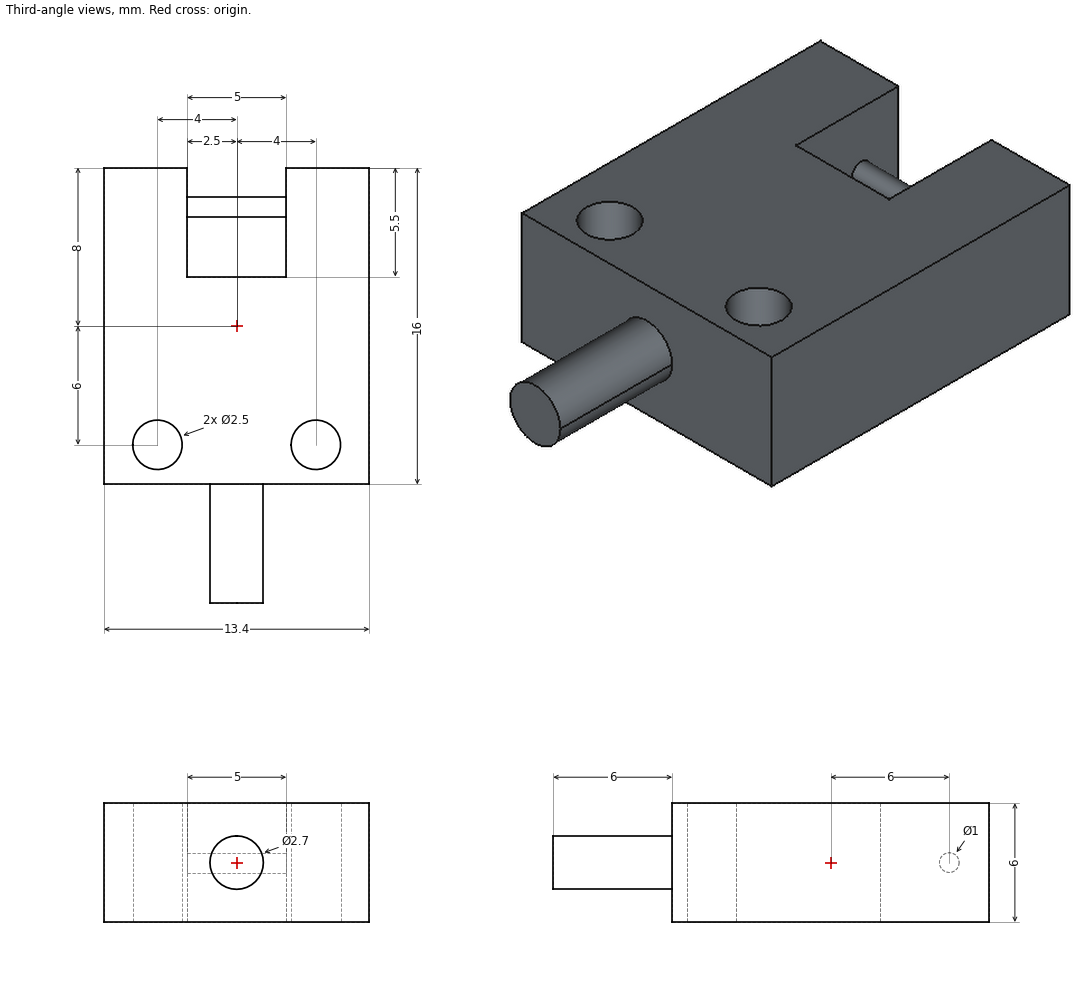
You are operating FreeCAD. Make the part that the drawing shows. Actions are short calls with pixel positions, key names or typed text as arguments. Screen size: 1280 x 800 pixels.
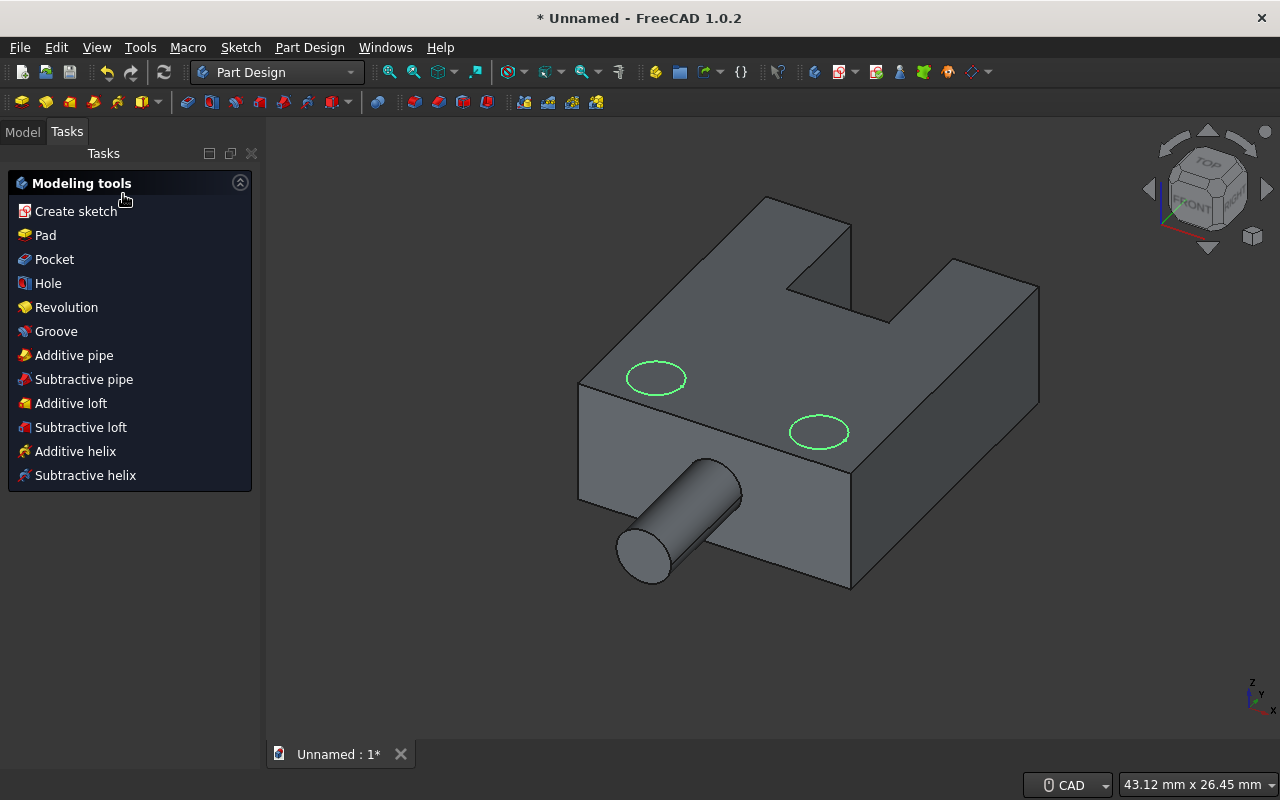
click(188, 102)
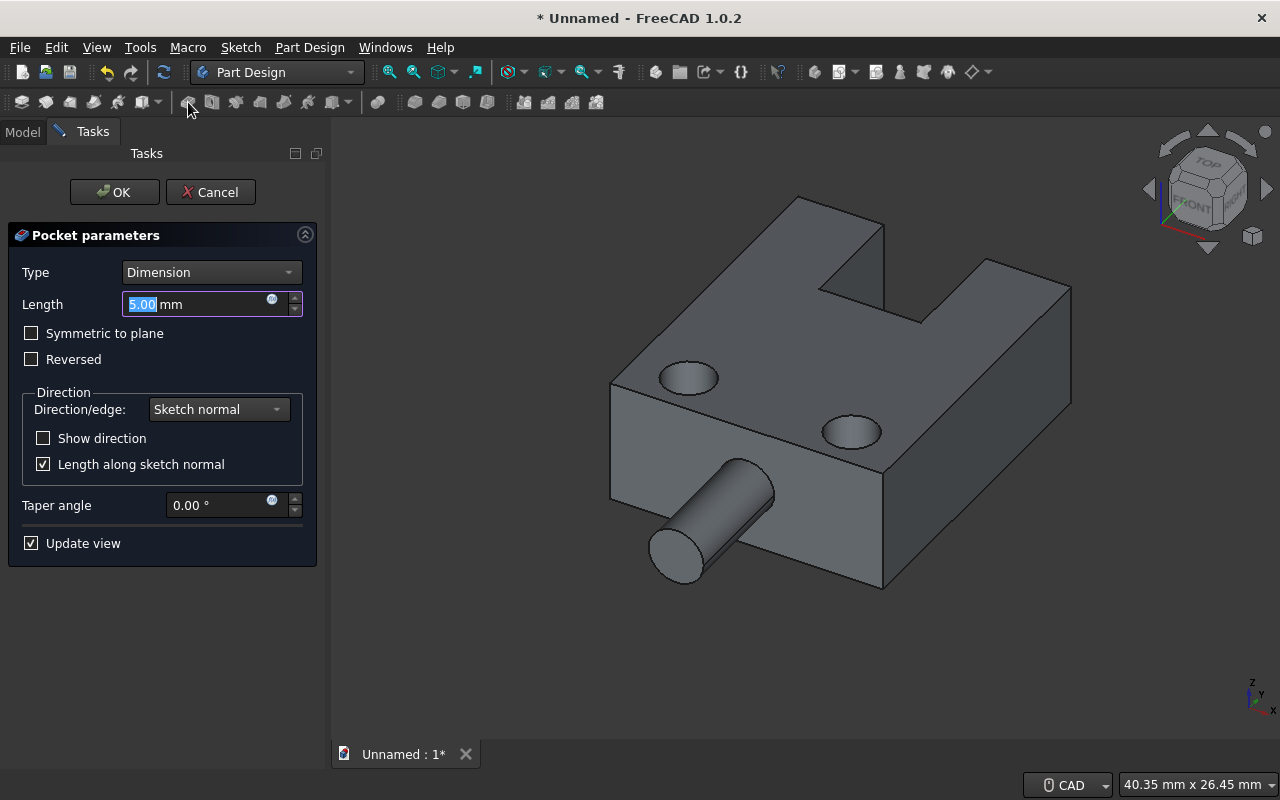
click(212, 272)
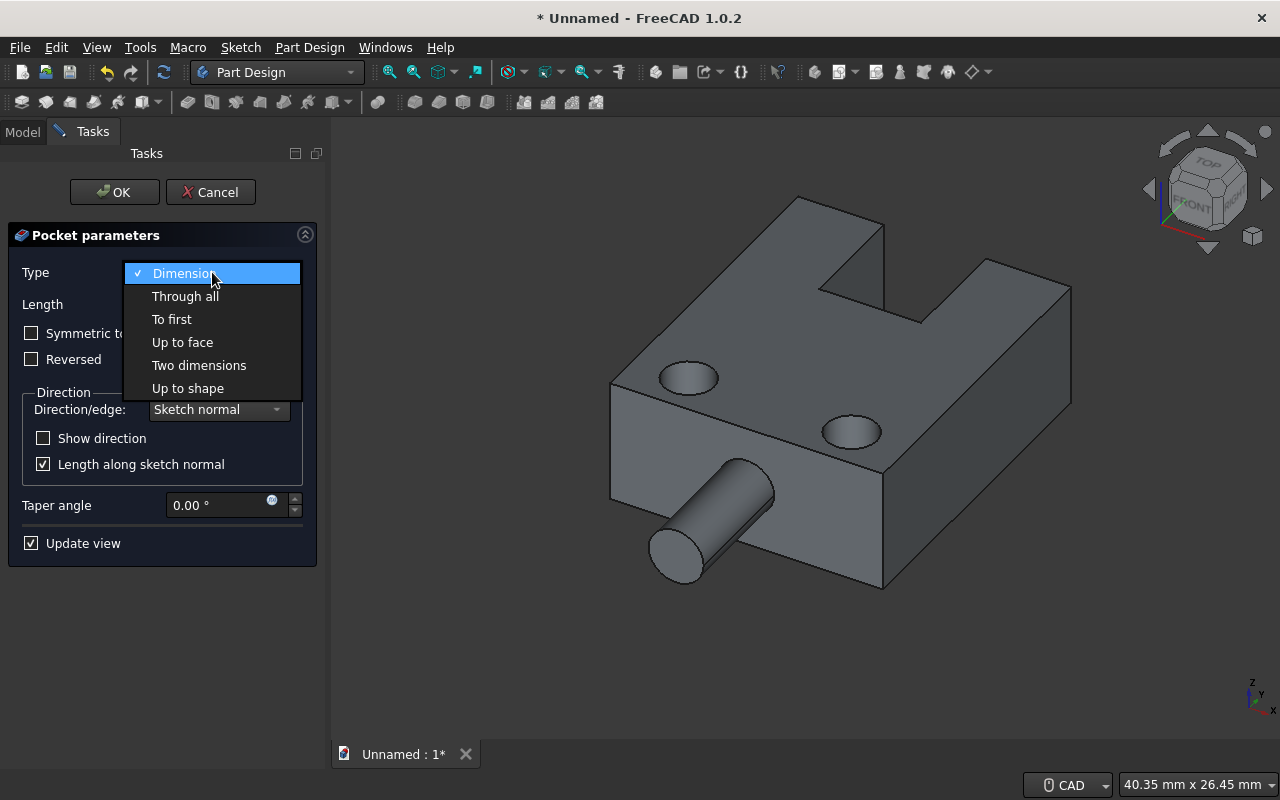
click(212, 296)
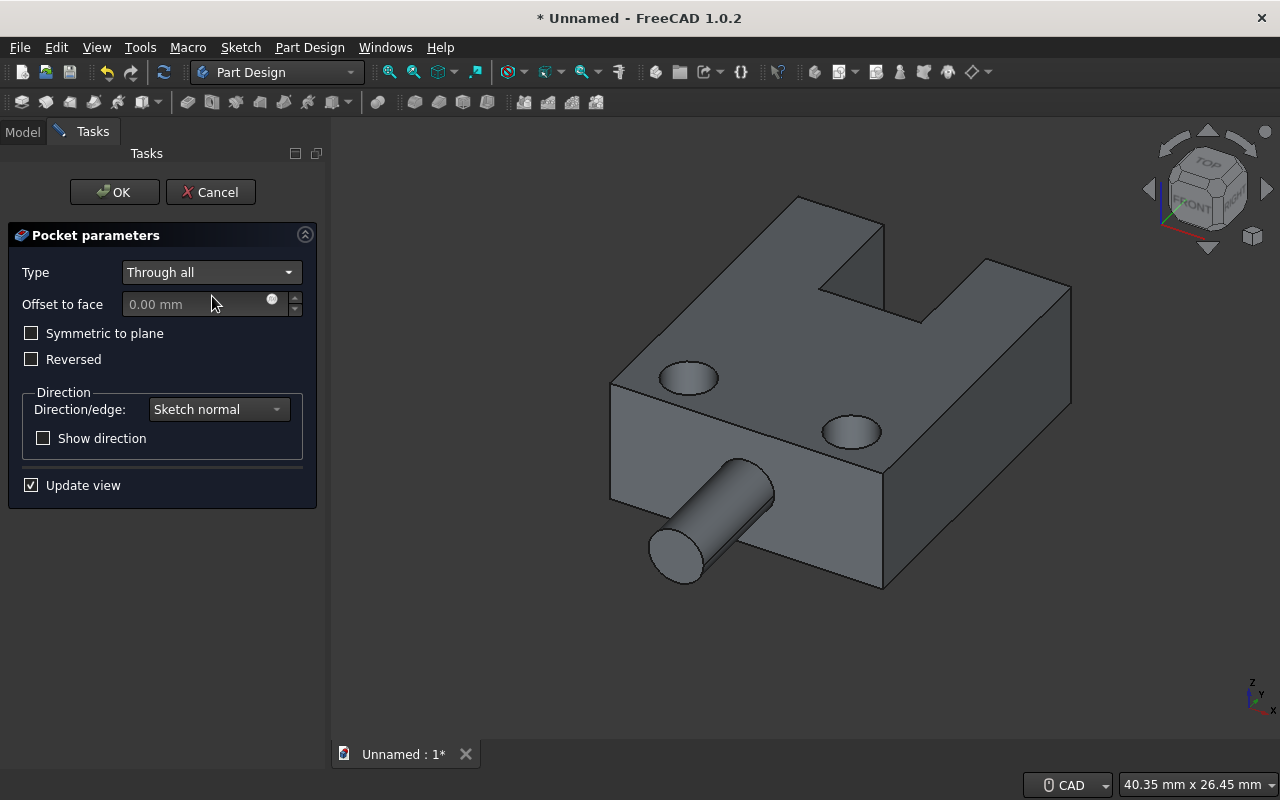
click(115, 192)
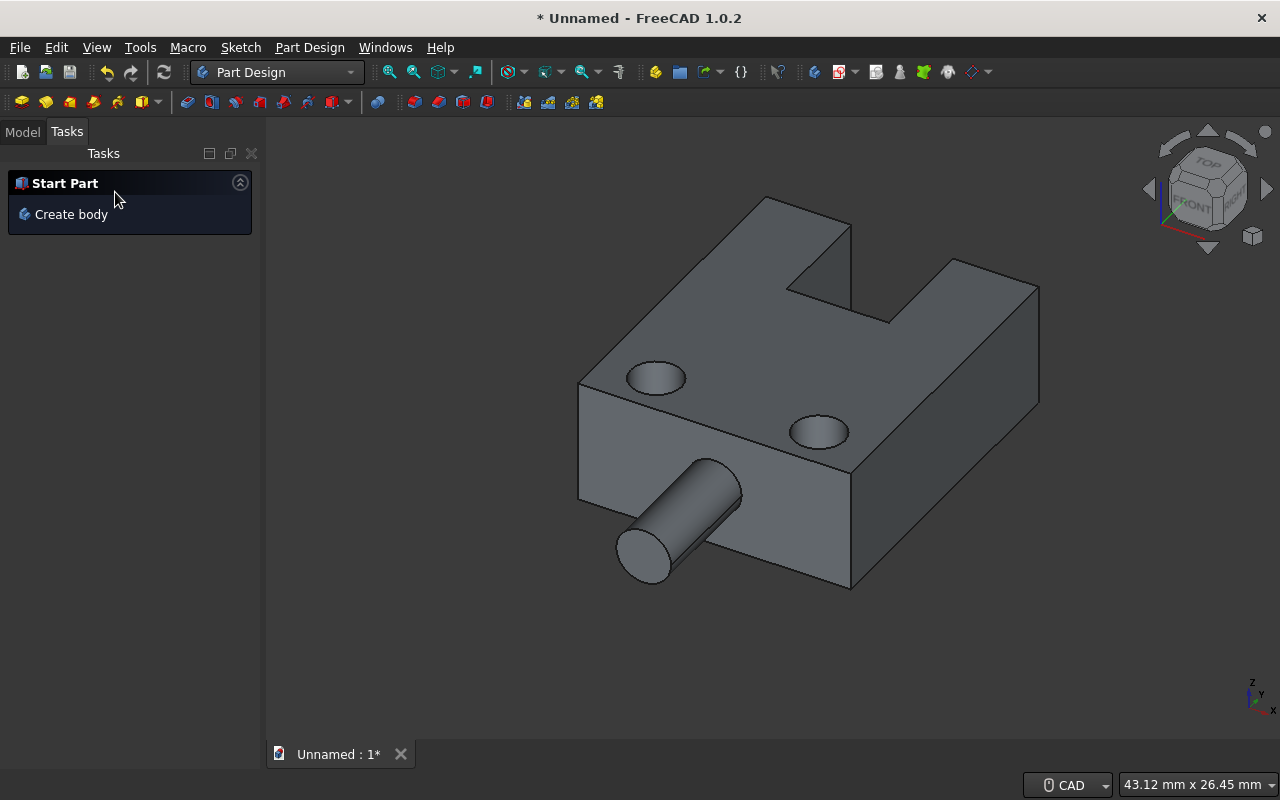
click(23, 131)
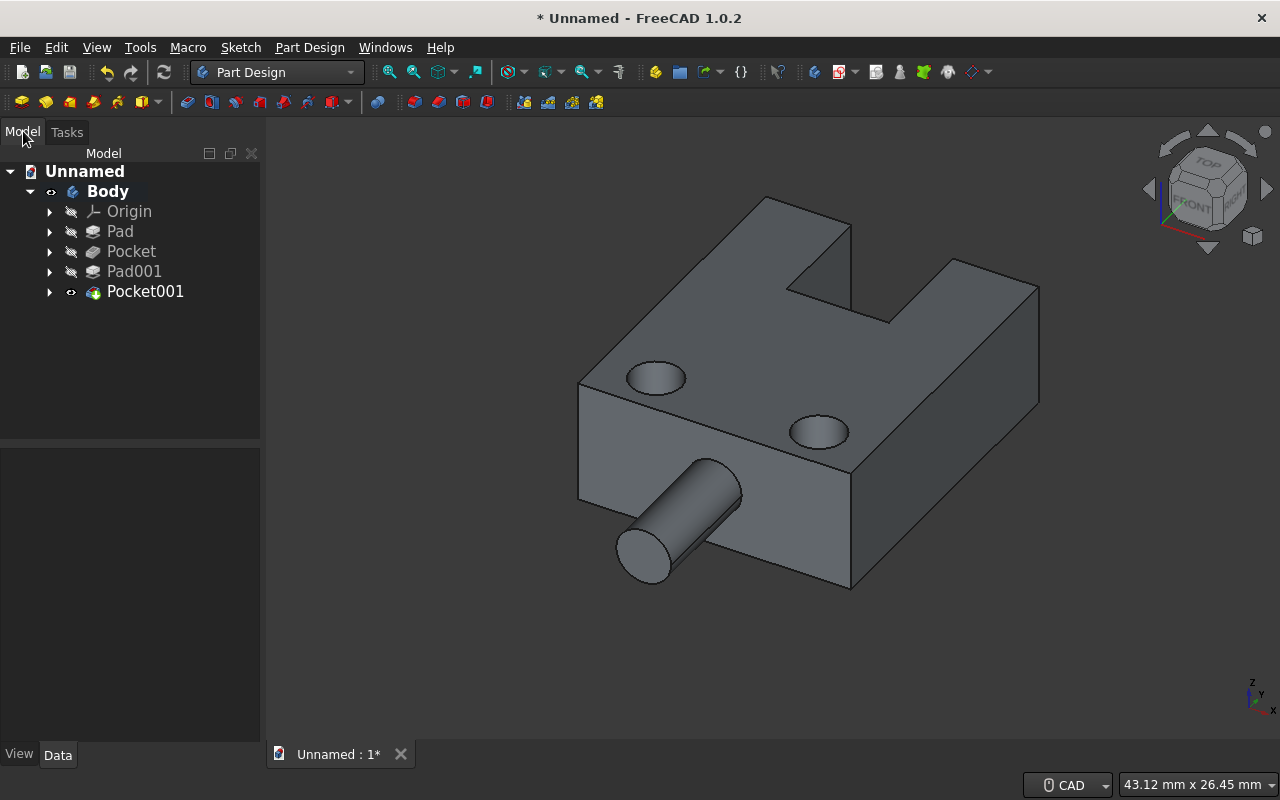
click(50, 212)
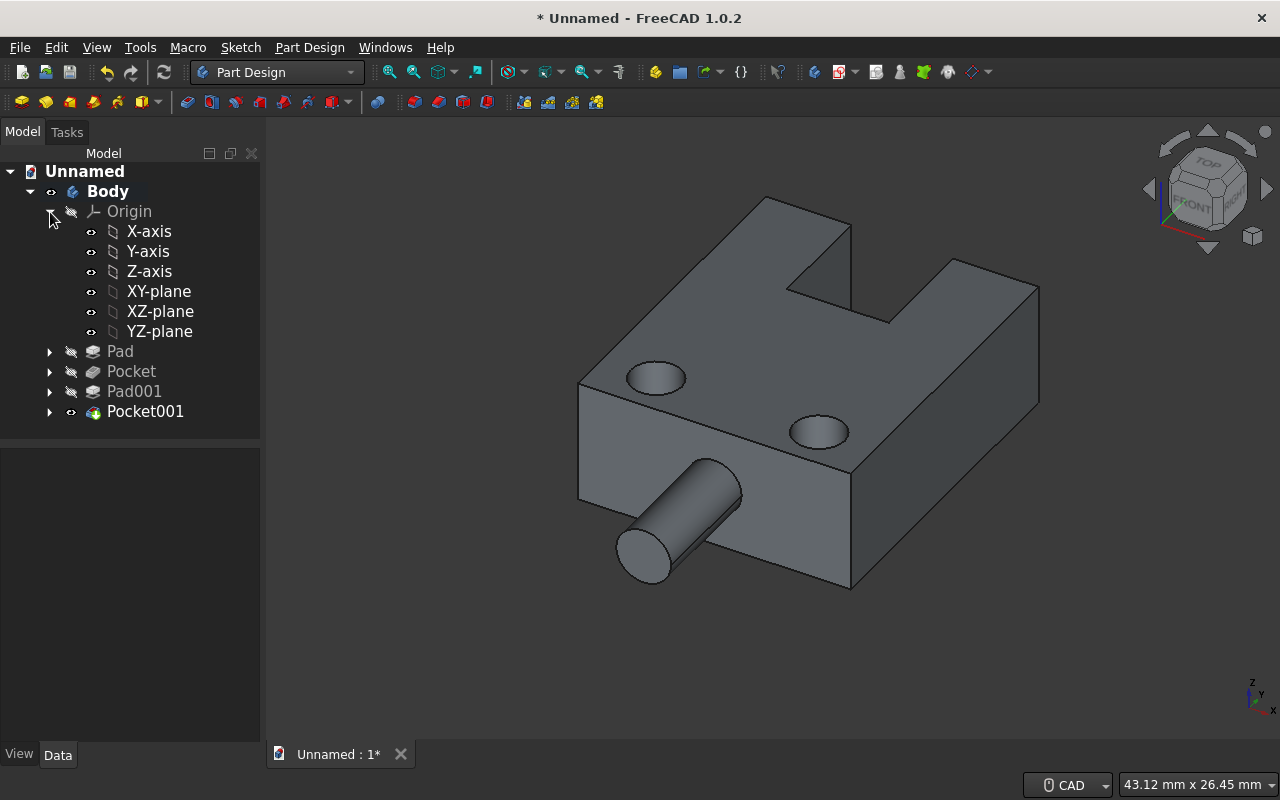
click(136, 332)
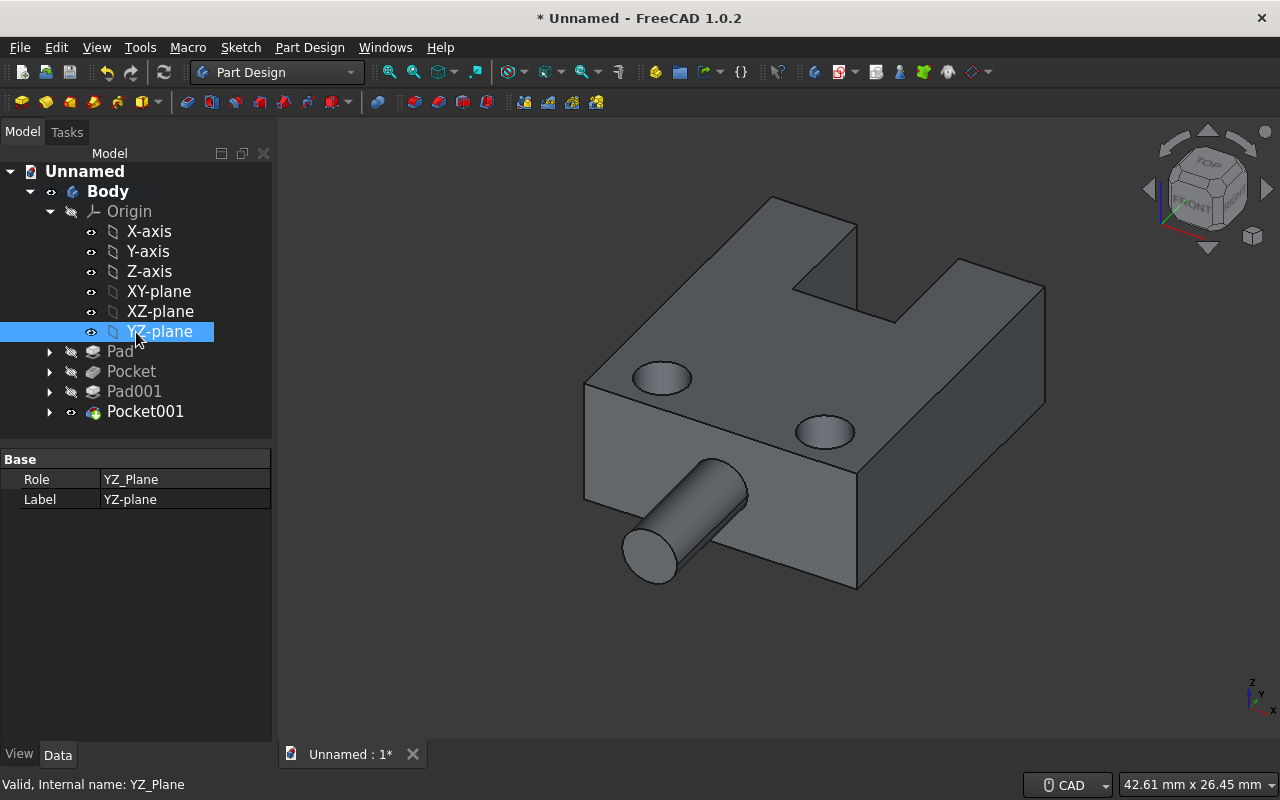
click(972, 72)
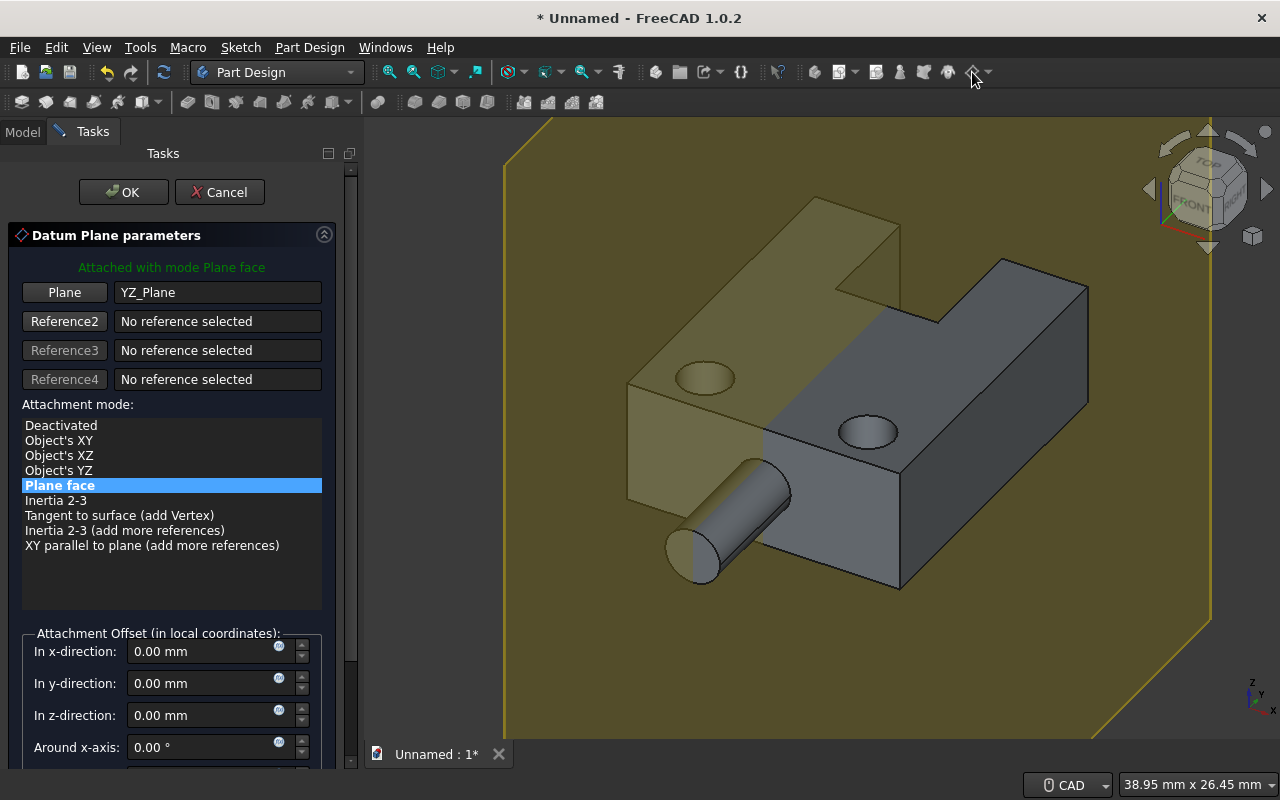
triple_click(210, 715)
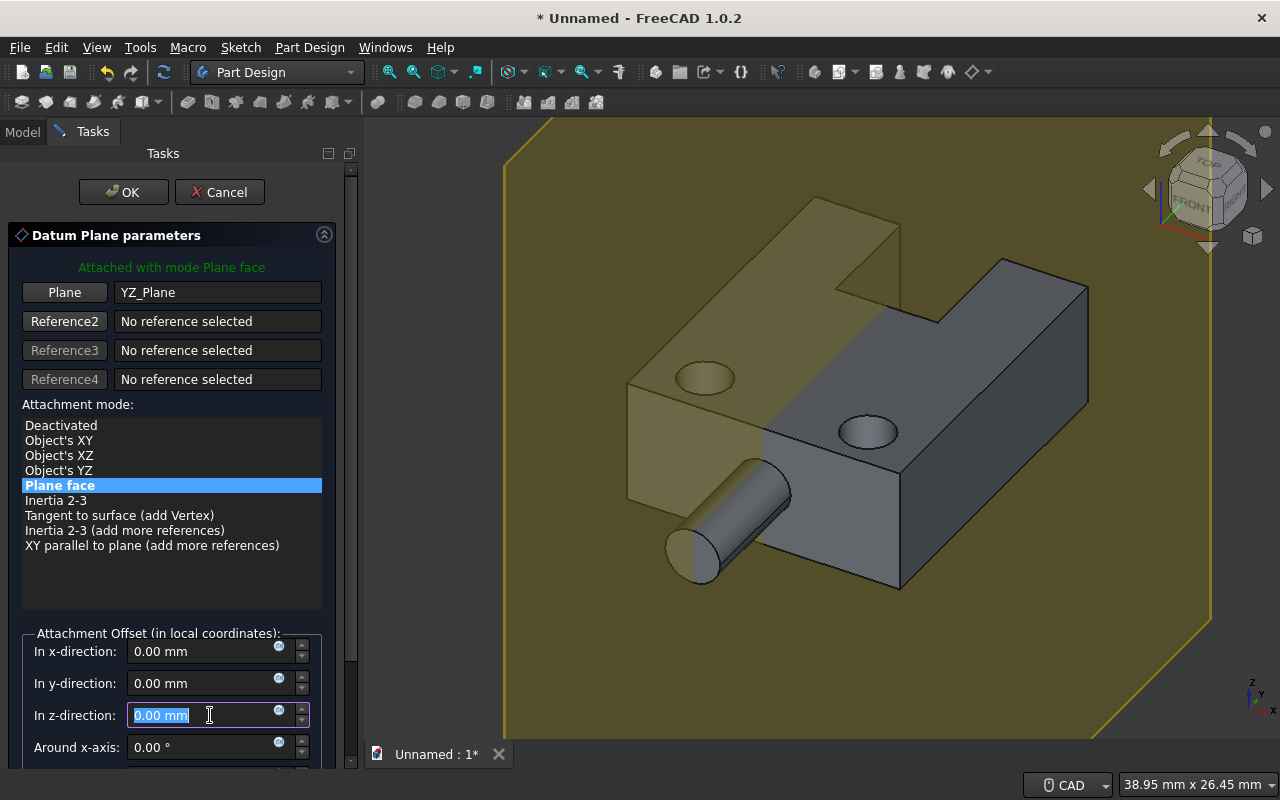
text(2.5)
key(Tab)